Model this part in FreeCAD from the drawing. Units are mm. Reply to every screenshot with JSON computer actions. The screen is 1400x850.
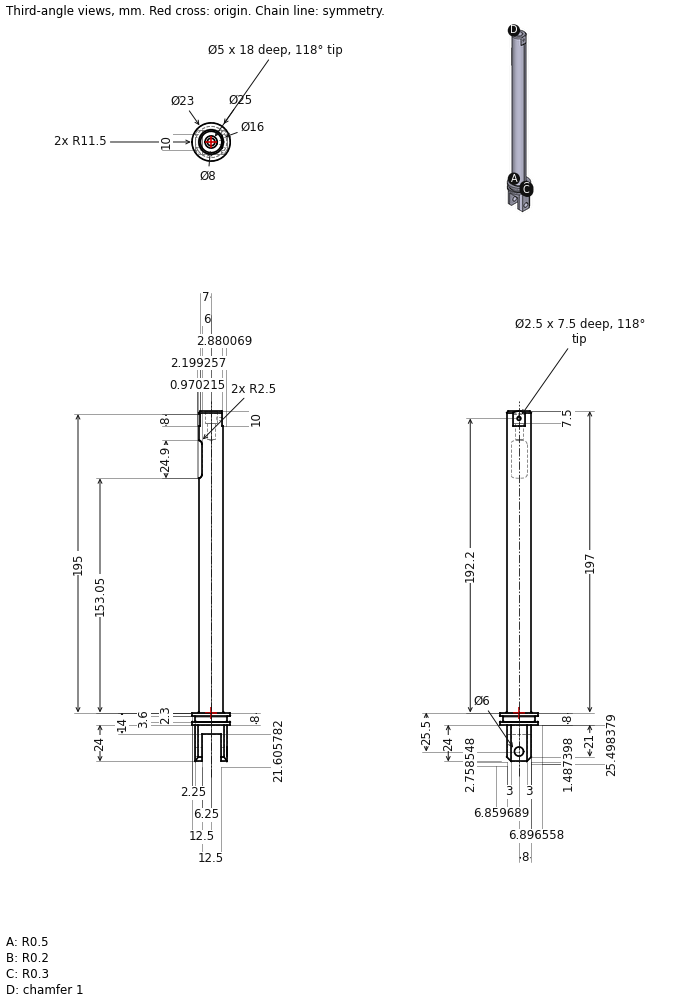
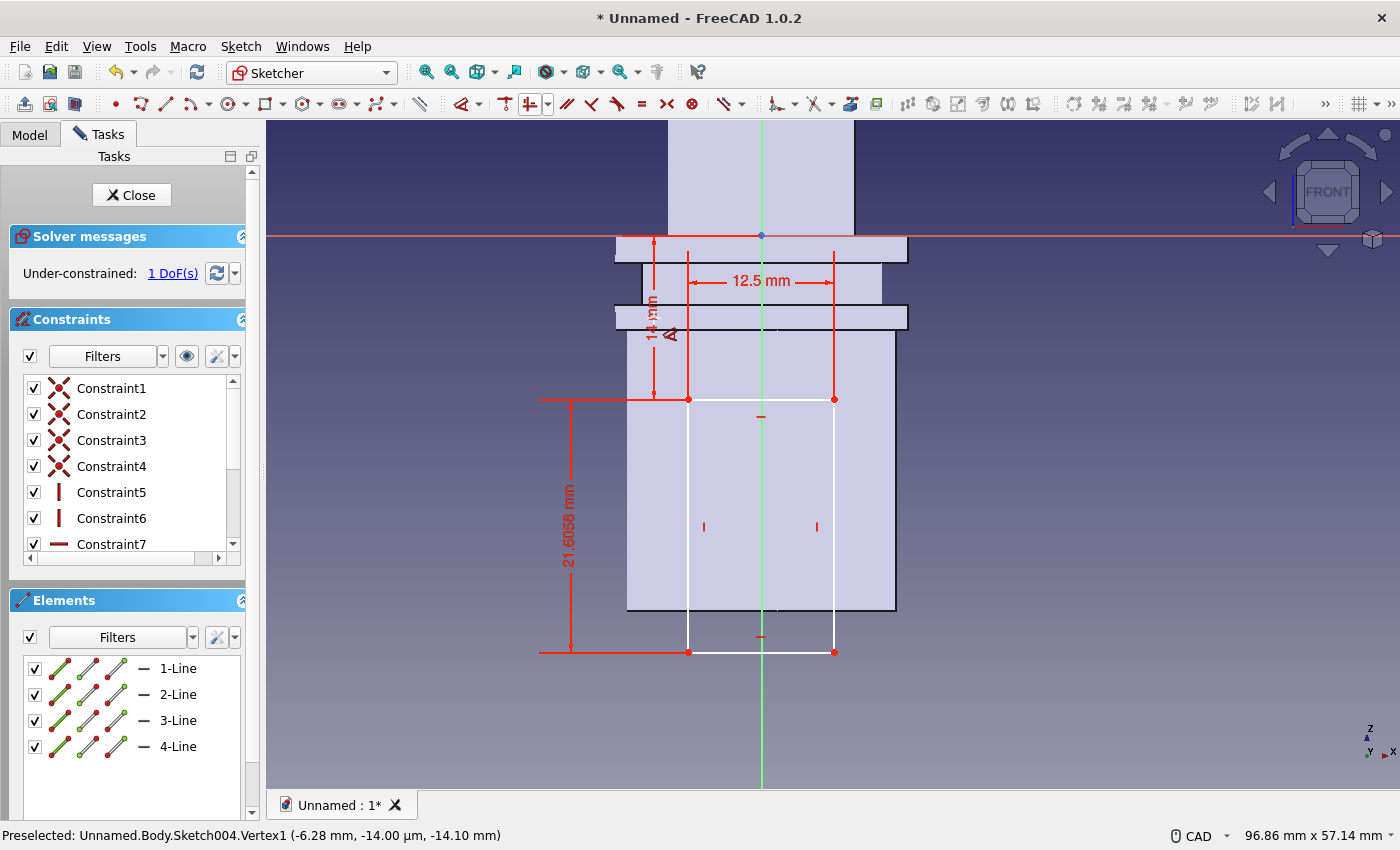
{"action": "left_click", "coordinate": [688, 400]}
{"action": "left_click", "coordinate": [725, 202]}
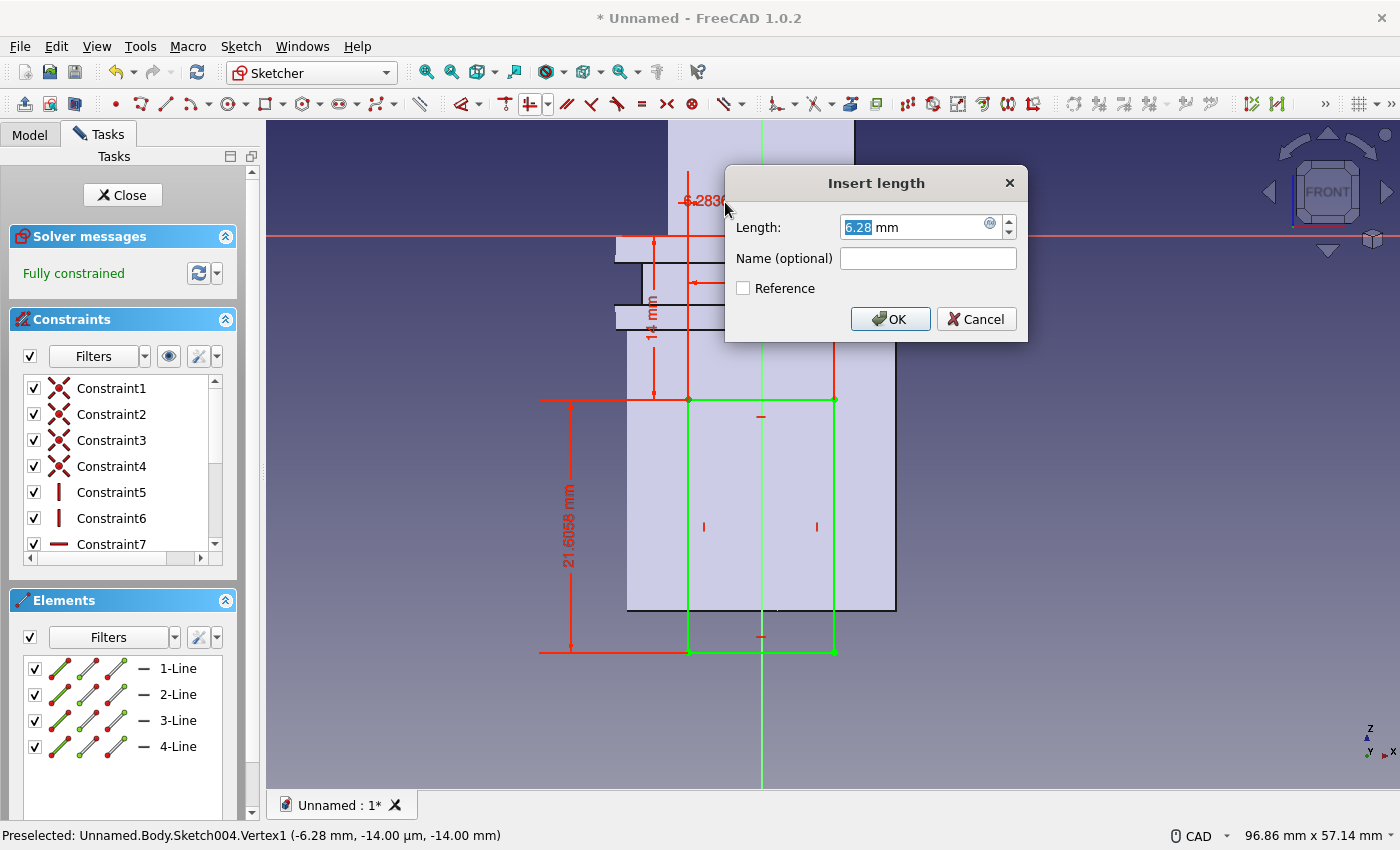
{"action": "type", "text": "6.25"}
{"action": "key", "text": "Return"}
{"action": "key", "text": "Escape"}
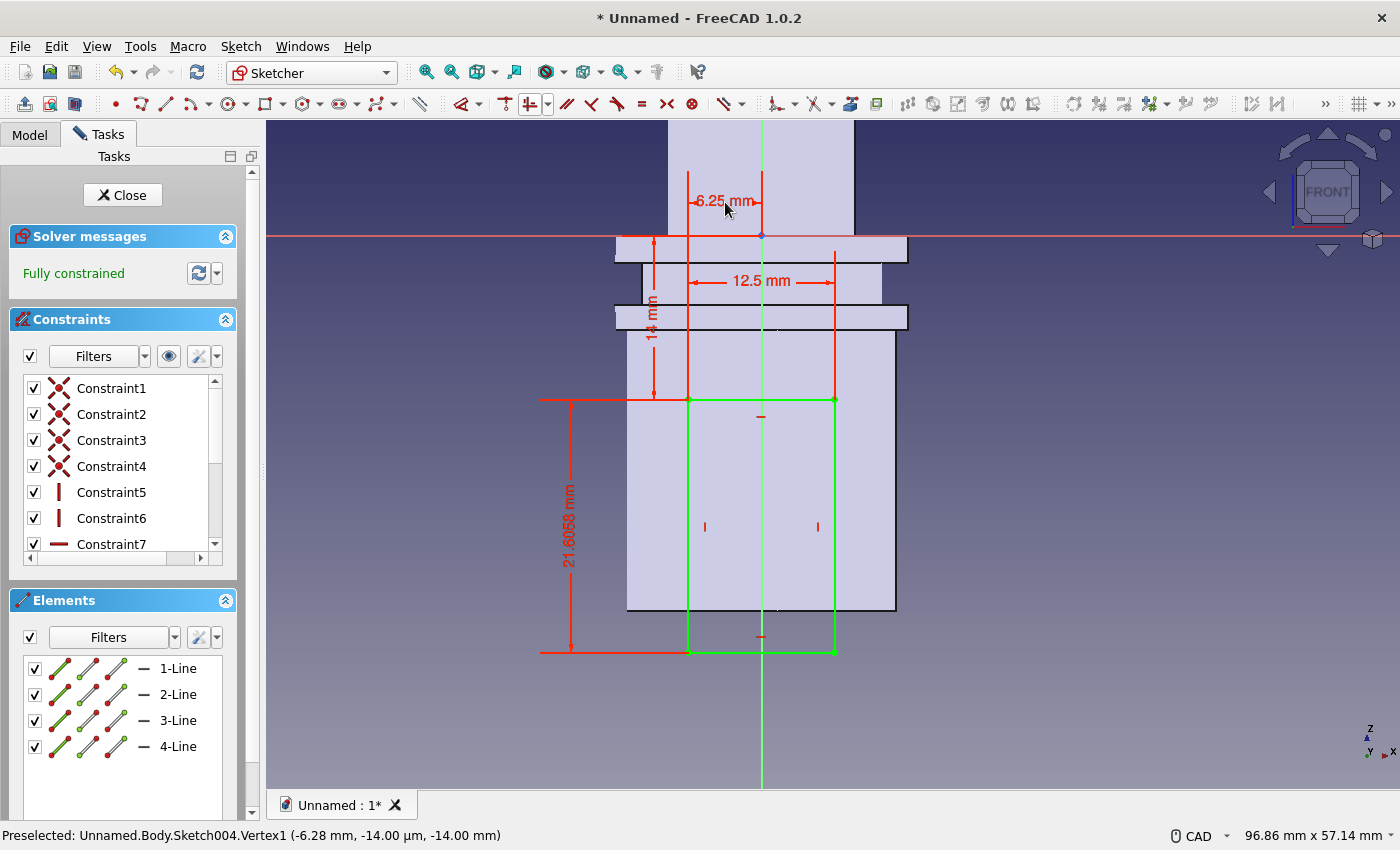
{"action": "left_click", "coordinate": [123, 195]}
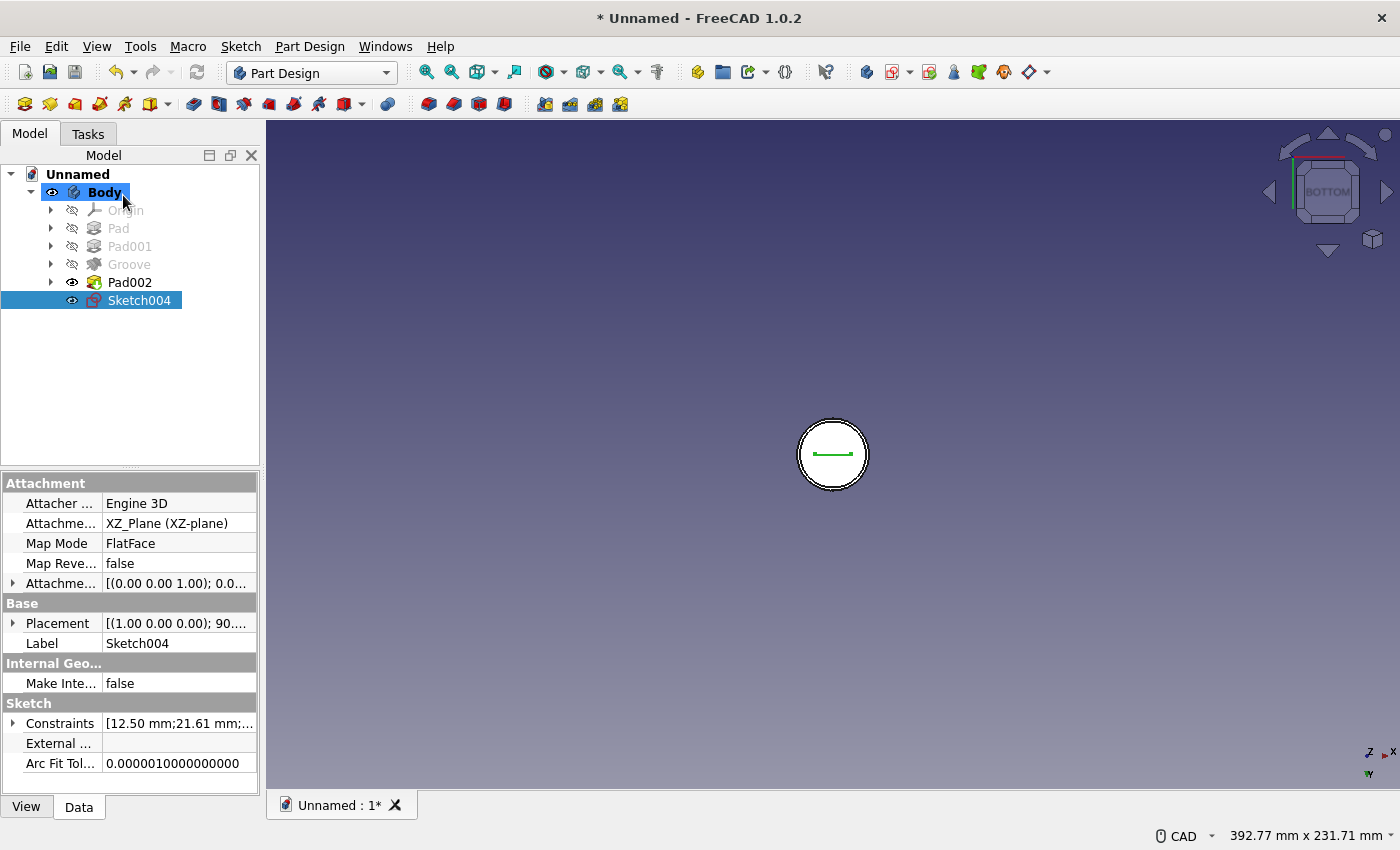
{"action": "left_click", "coordinate": [194, 104]}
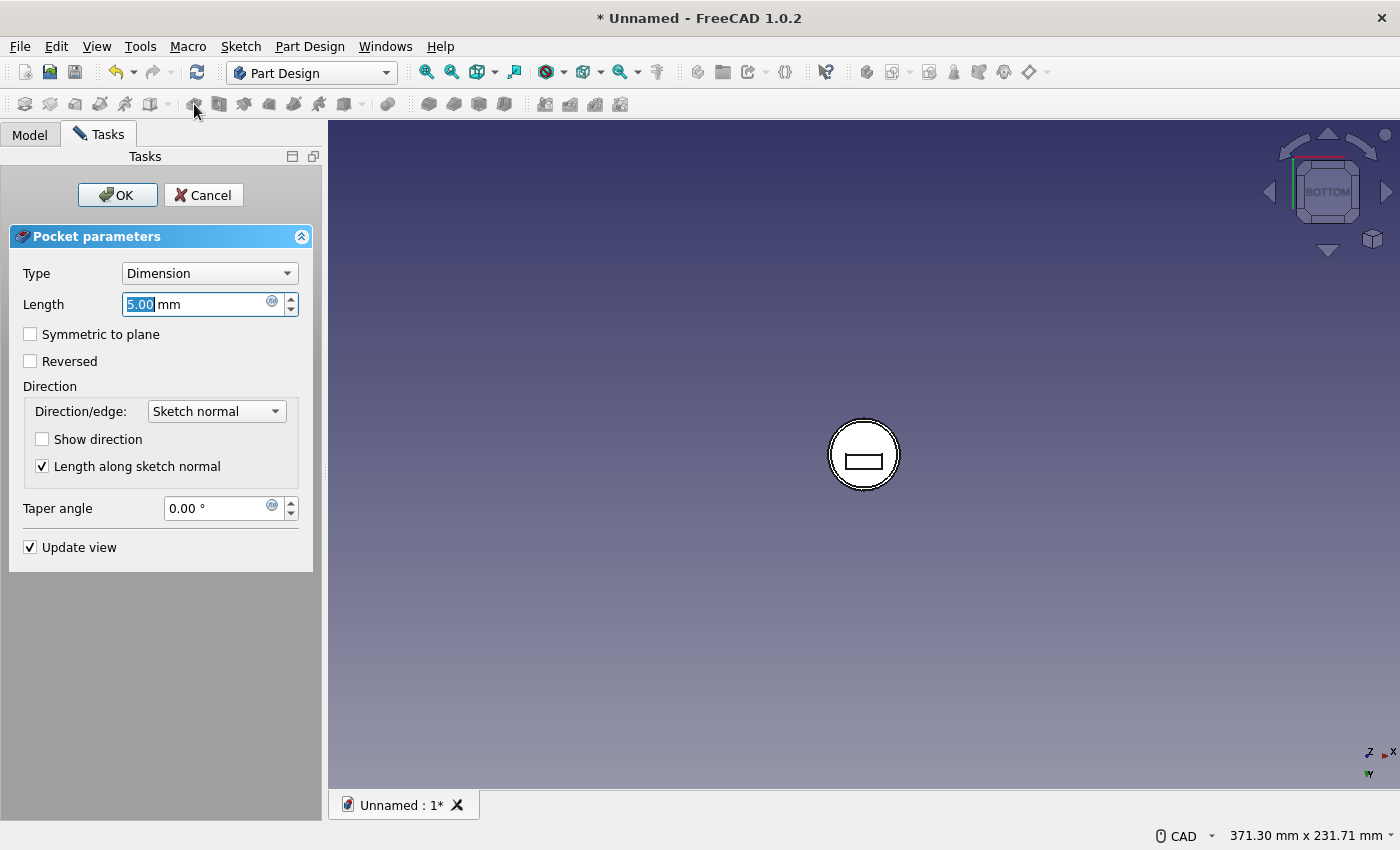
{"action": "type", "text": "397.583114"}
{"action": "key", "text": "Tab"}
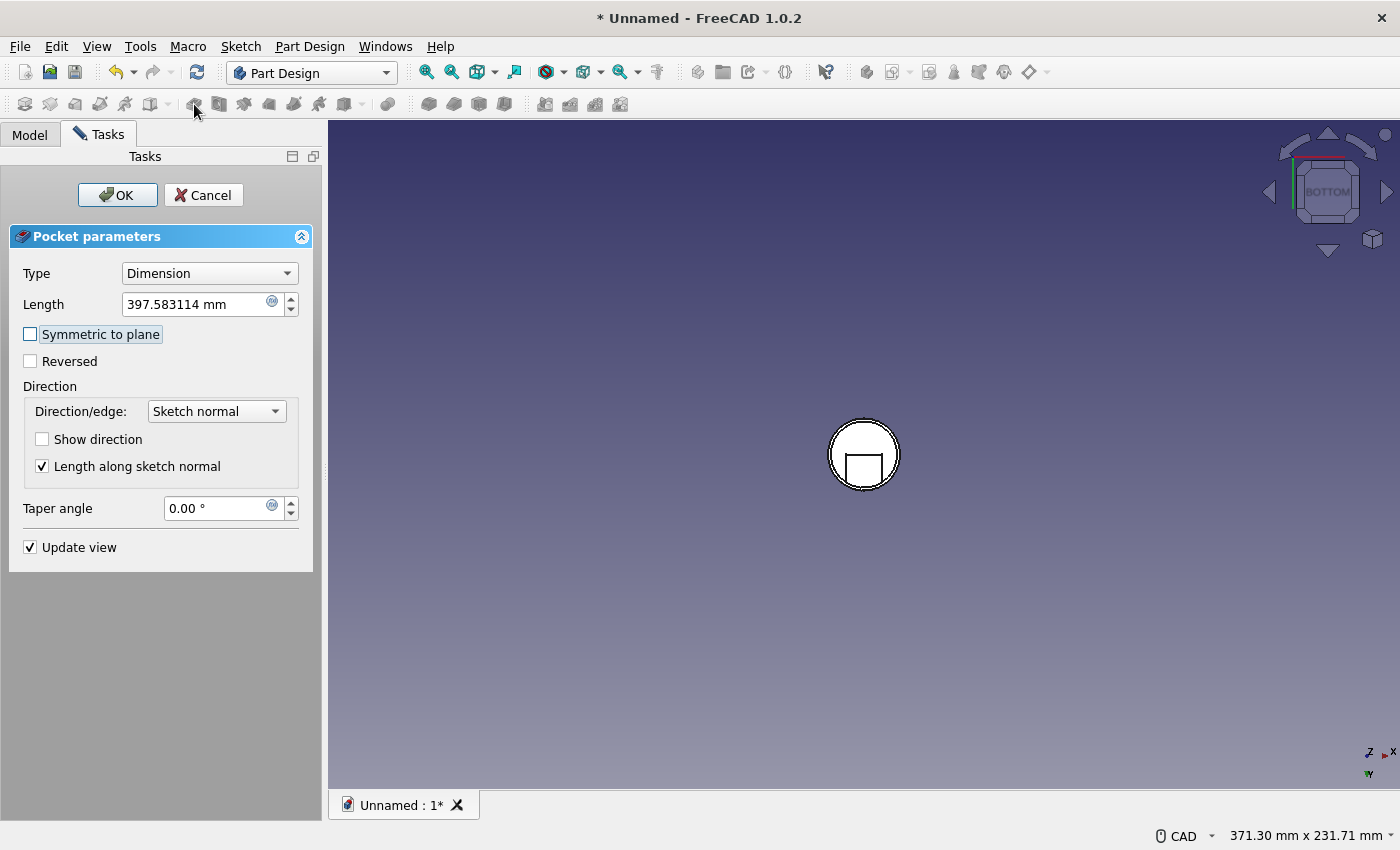
{"action": "left_click", "coordinate": [31, 334]}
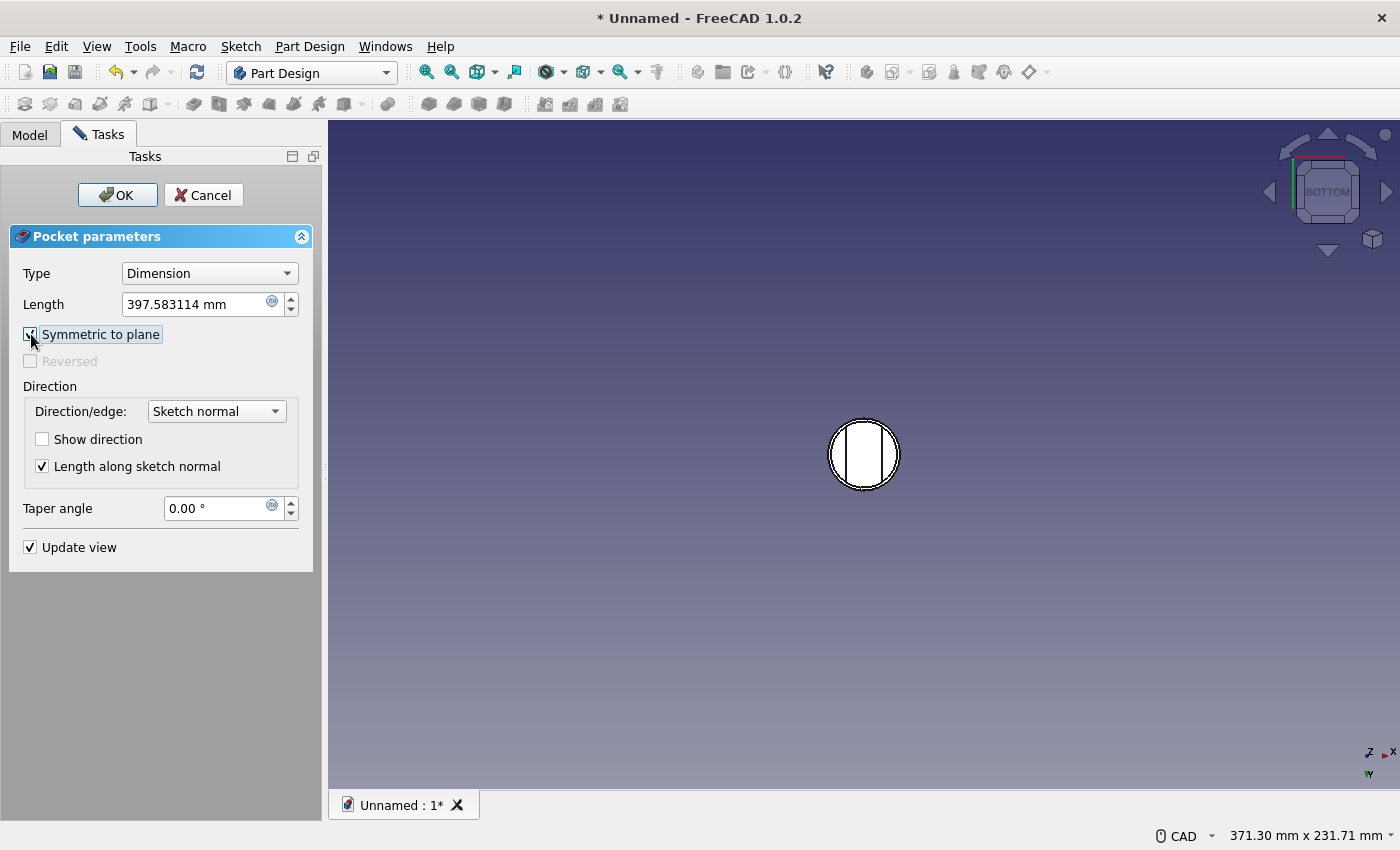
{"action": "left_click", "coordinate": [118, 195]}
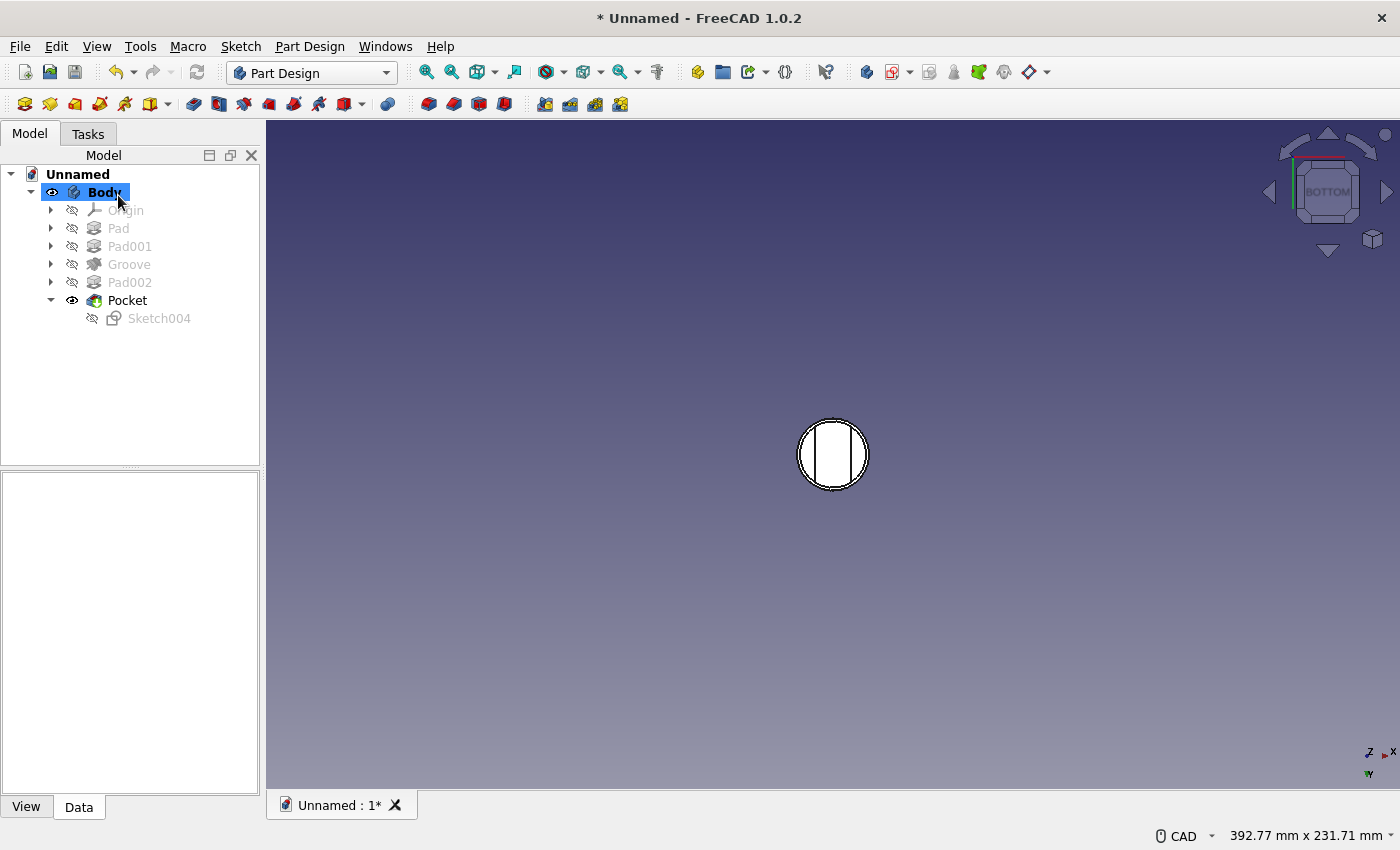
{"action": "left_click", "coordinate": [427, 72]}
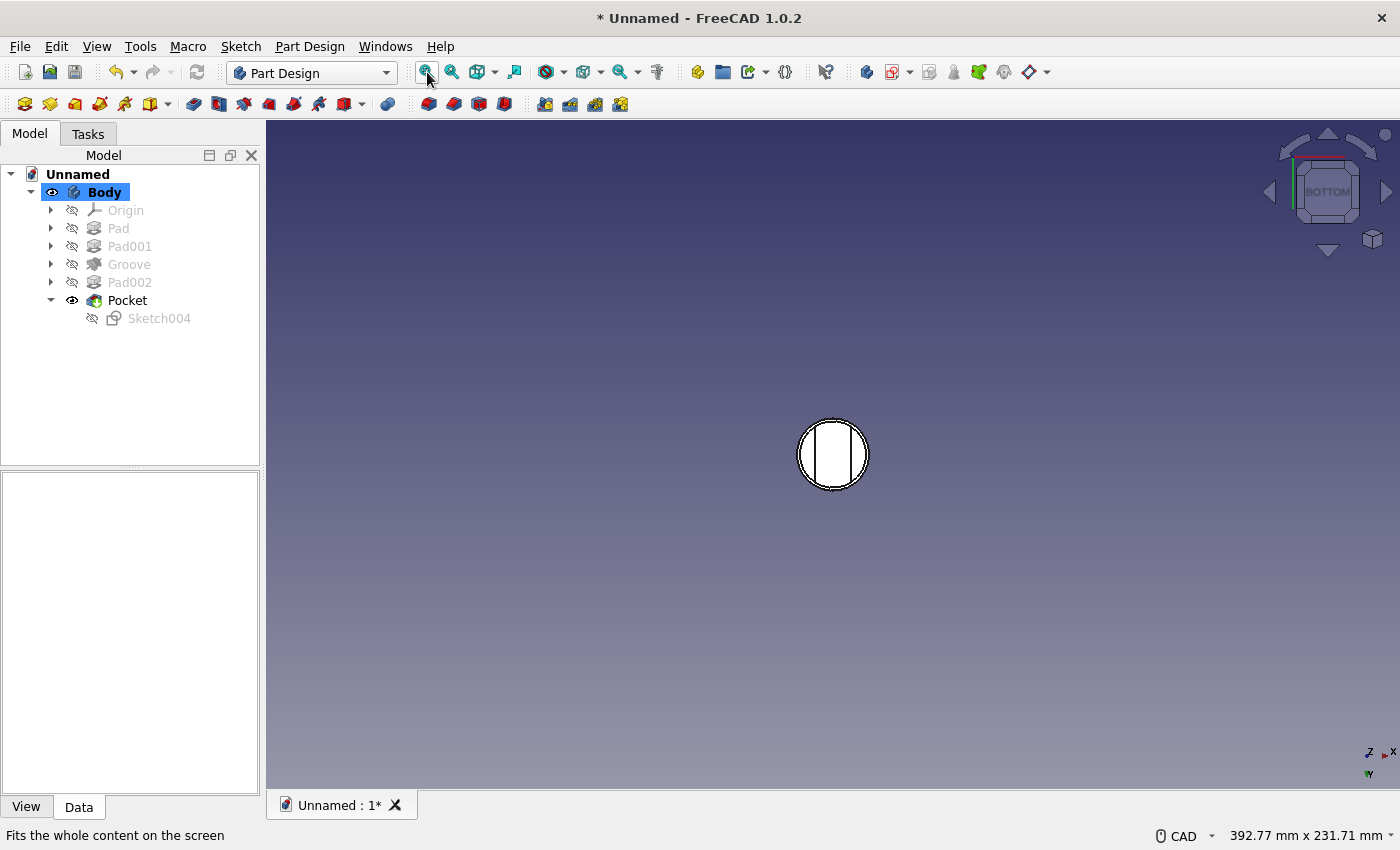
{"action": "left_click", "coordinate": [892, 72]}